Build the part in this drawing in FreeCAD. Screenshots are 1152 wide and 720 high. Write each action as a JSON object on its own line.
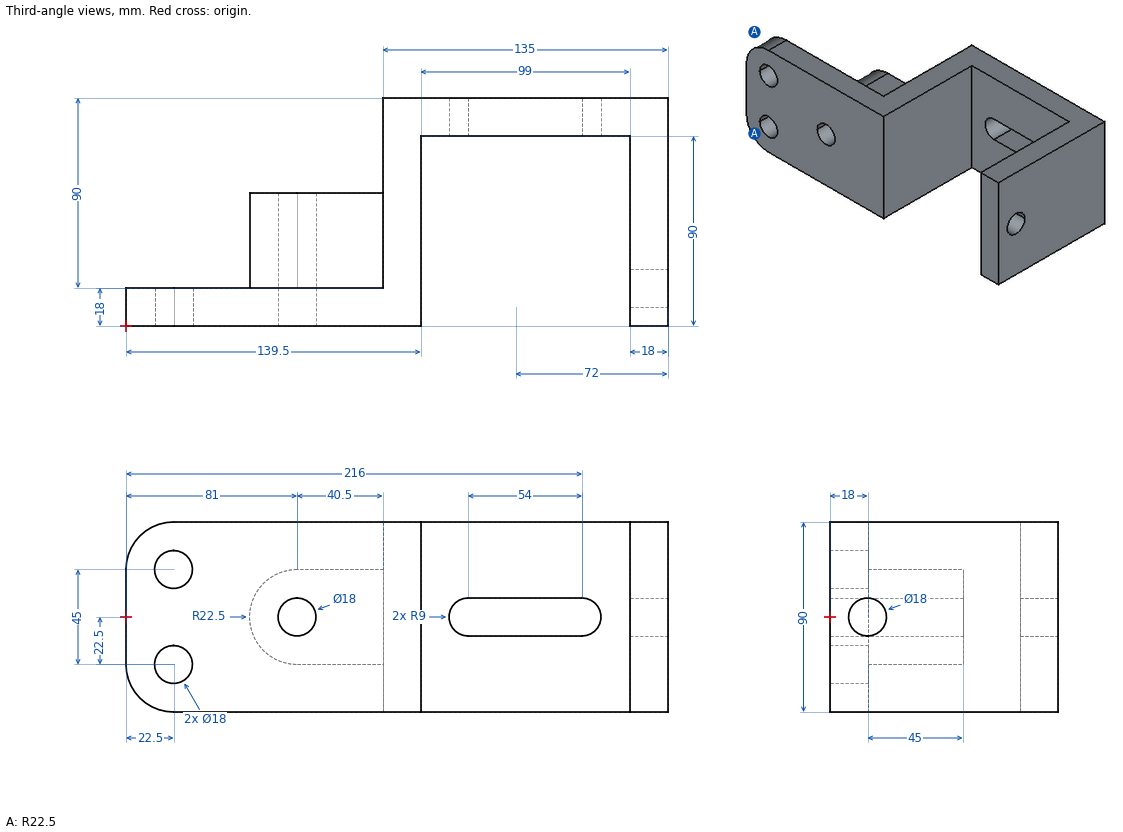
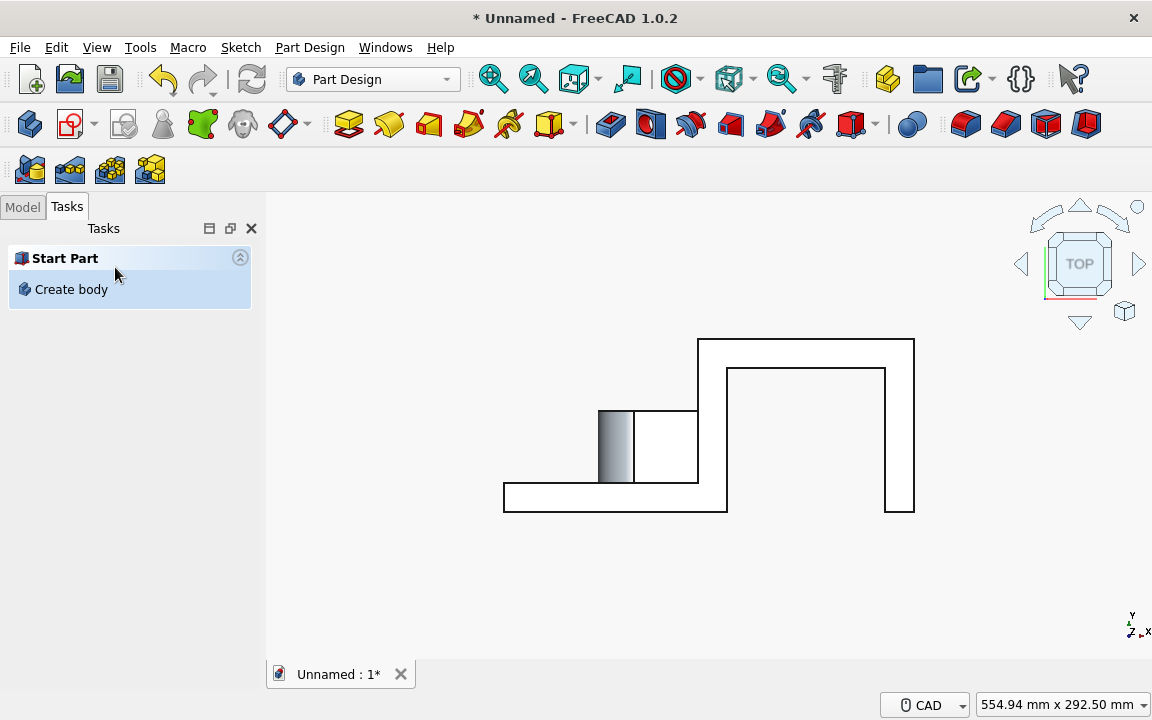
{"action": "left_click", "coordinate": [504, 496]}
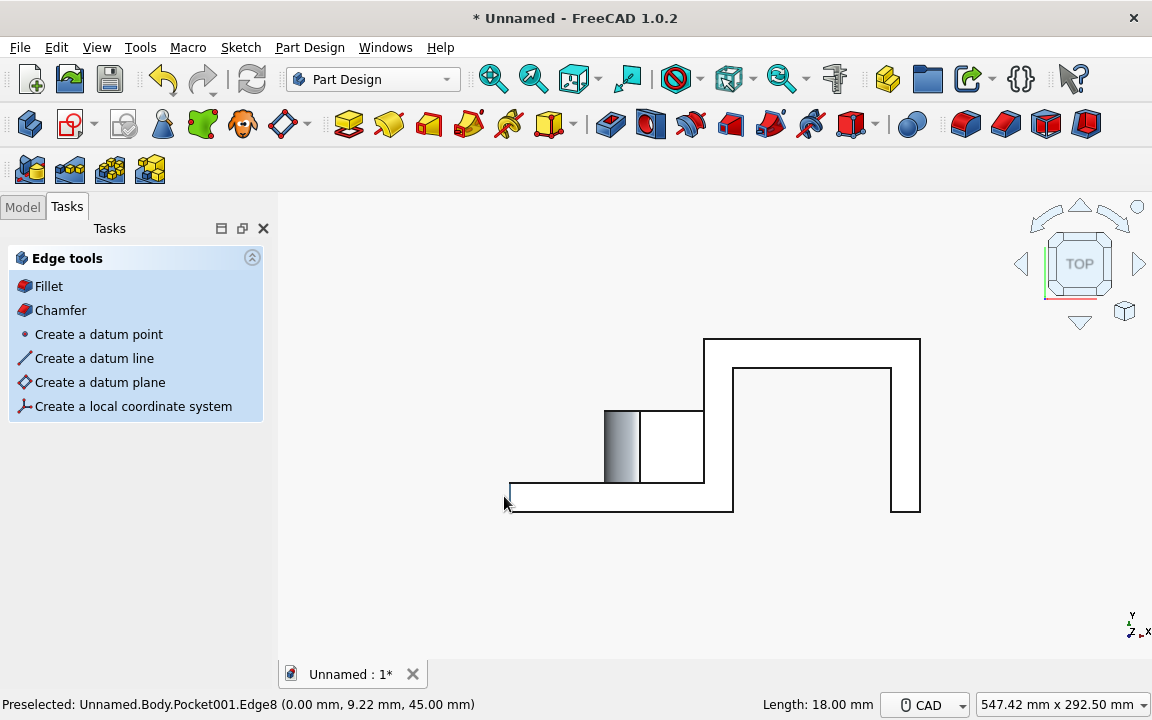
{"action": "key", "text": "1"}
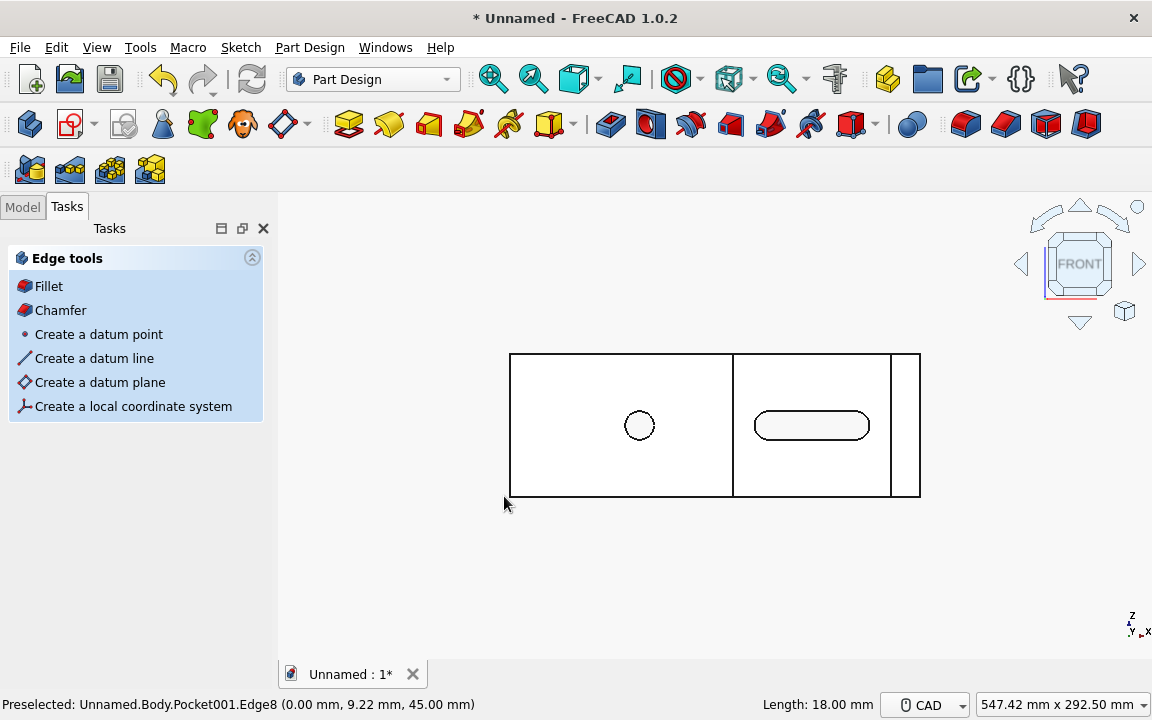
{"action": "key", "text": "3"}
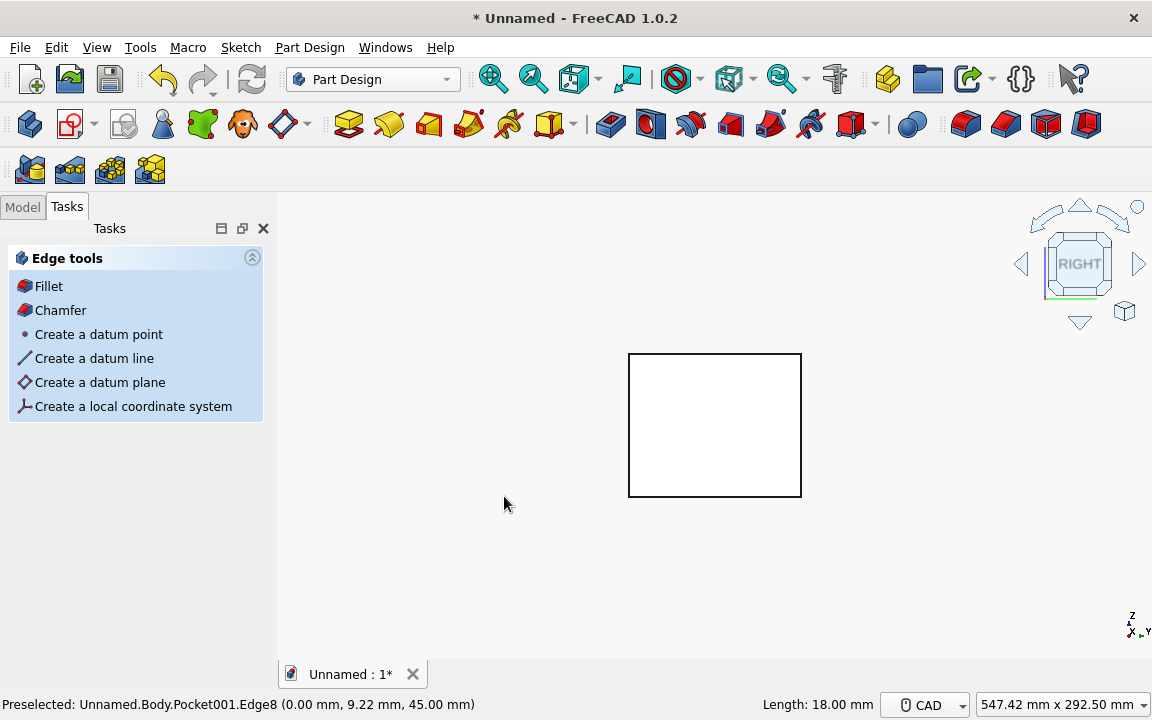
{"action": "left_click", "coordinate": [494, 80]}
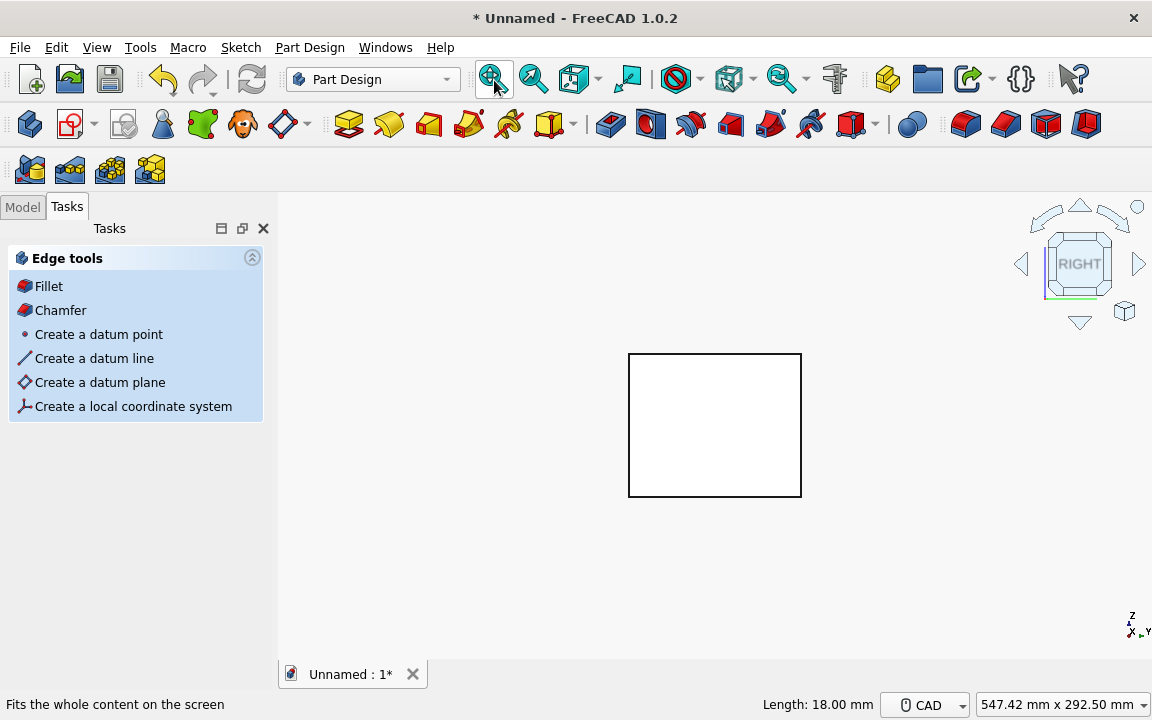
{"action": "key", "text": "5"}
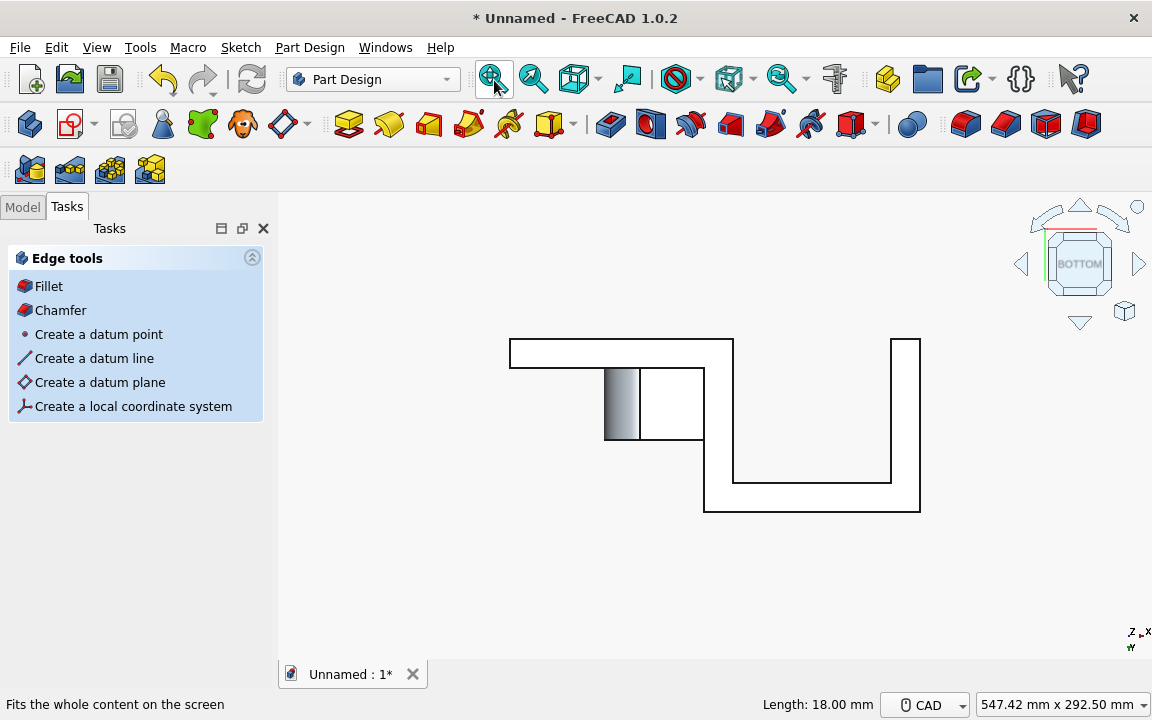
{"action": "left_click", "coordinate": [510, 353], "text": "ctrl"}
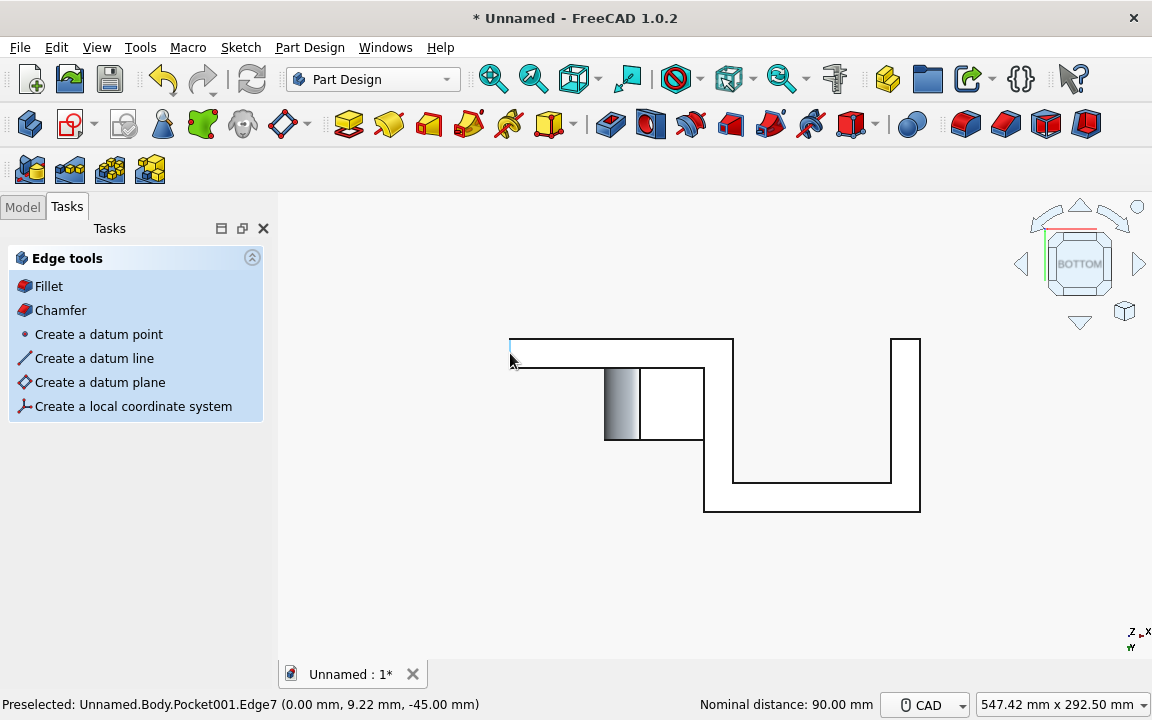
{"action": "left_click", "coordinate": [966, 124]}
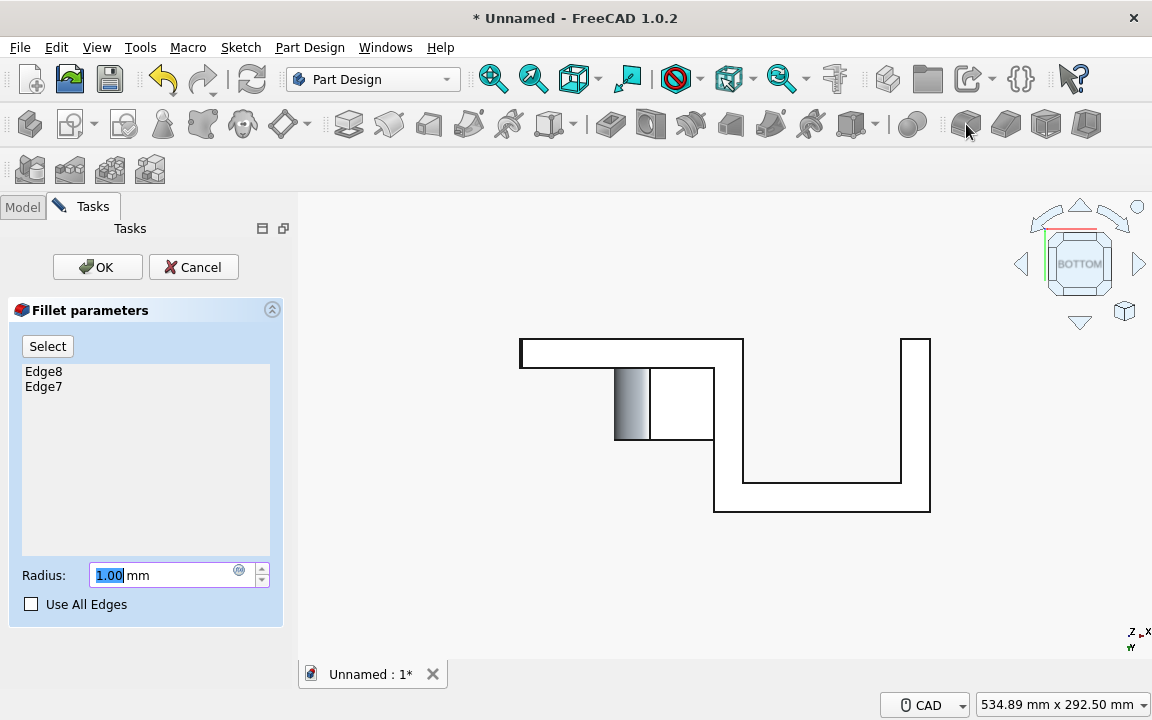
{"action": "type", "text": "22.5"}
{"action": "key", "text": "Tab"}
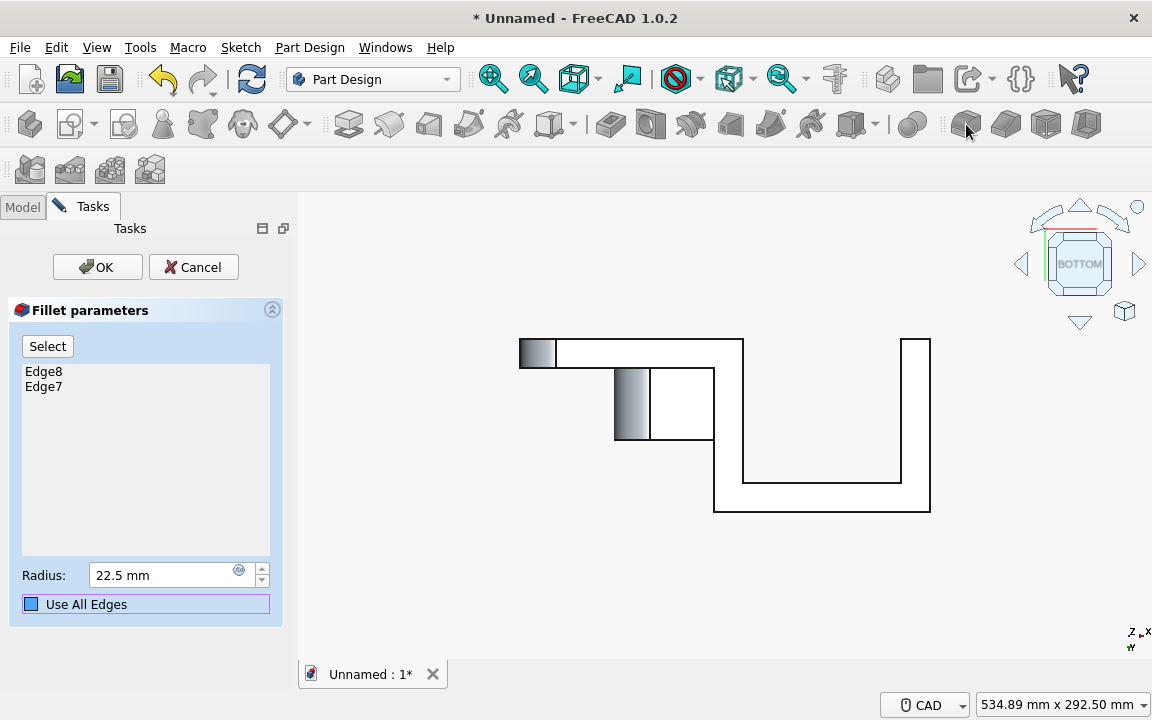
{"action": "left_click", "coordinate": [98, 267]}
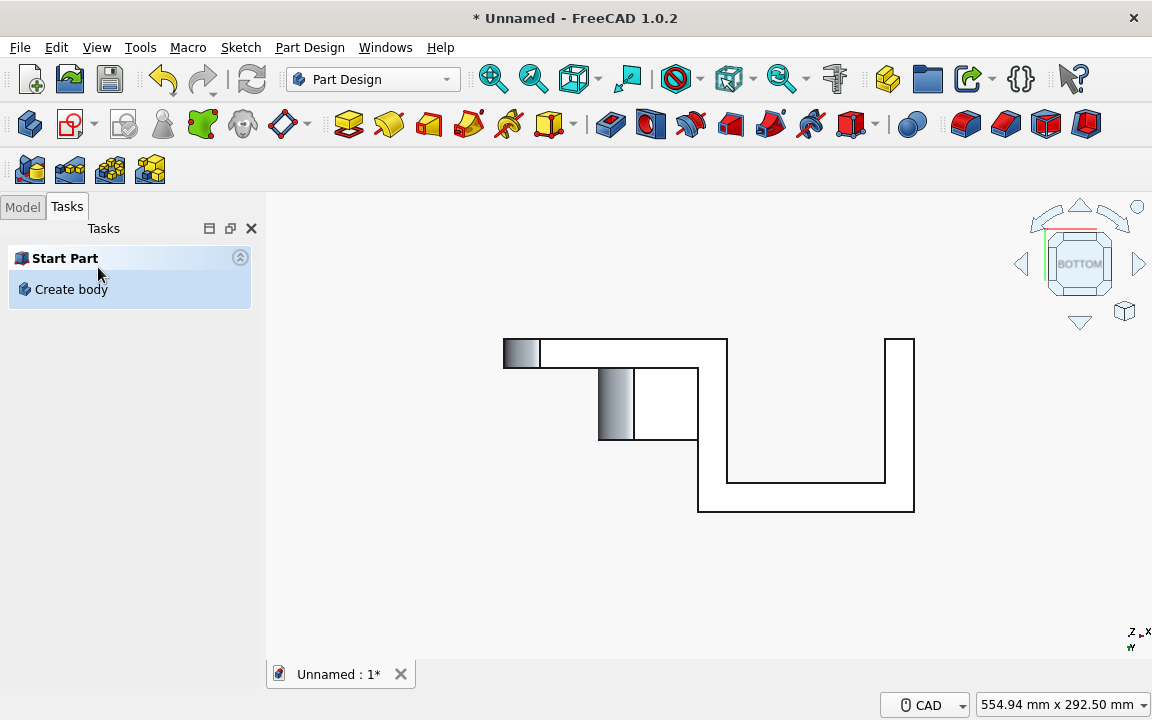
{"action": "key", "text": "4"}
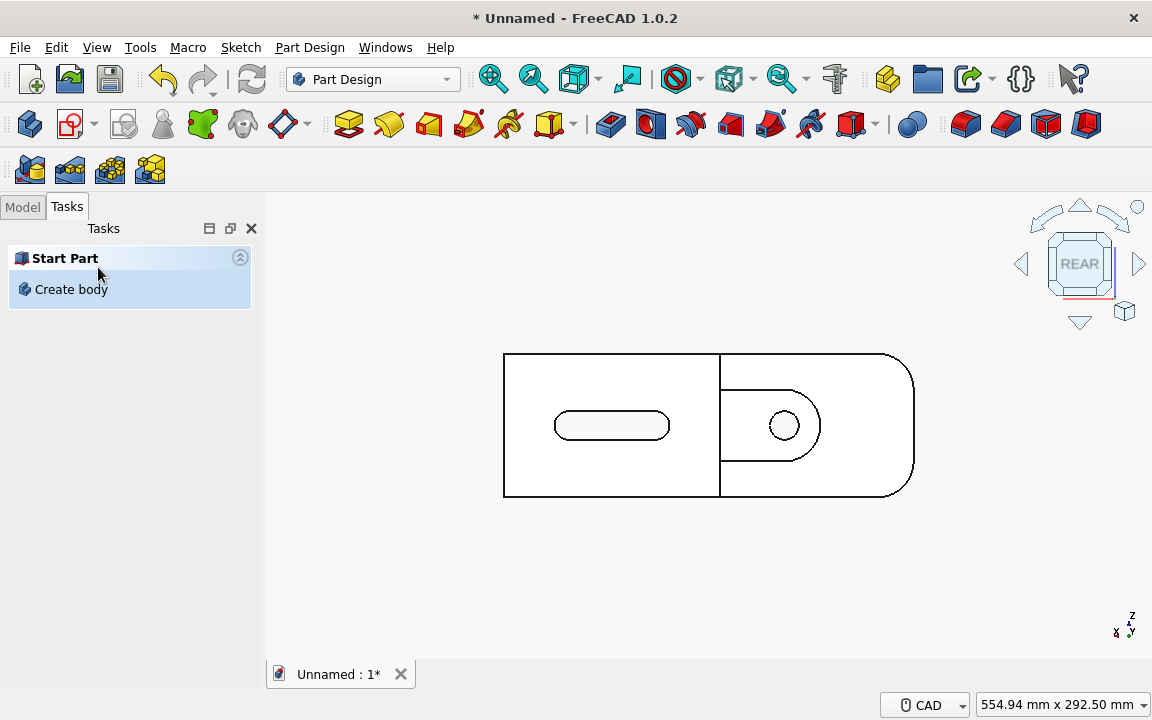
{"action": "left_click", "coordinate": [872, 404]}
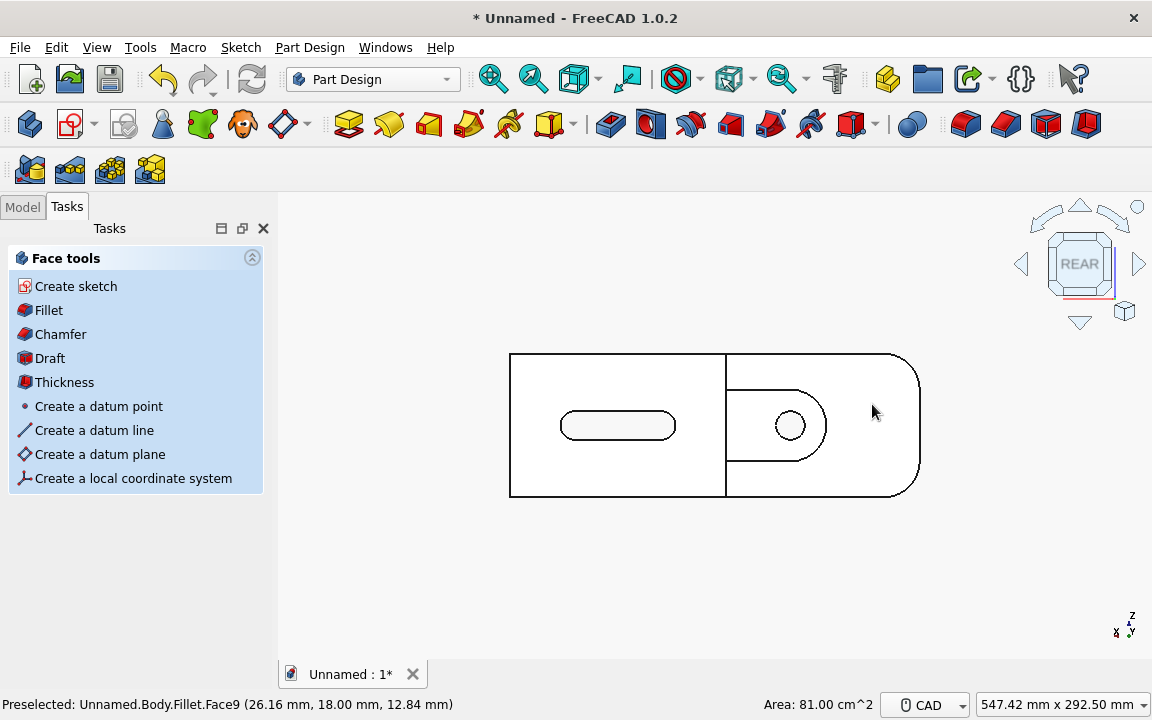
{"action": "left_click", "coordinate": [70, 124]}